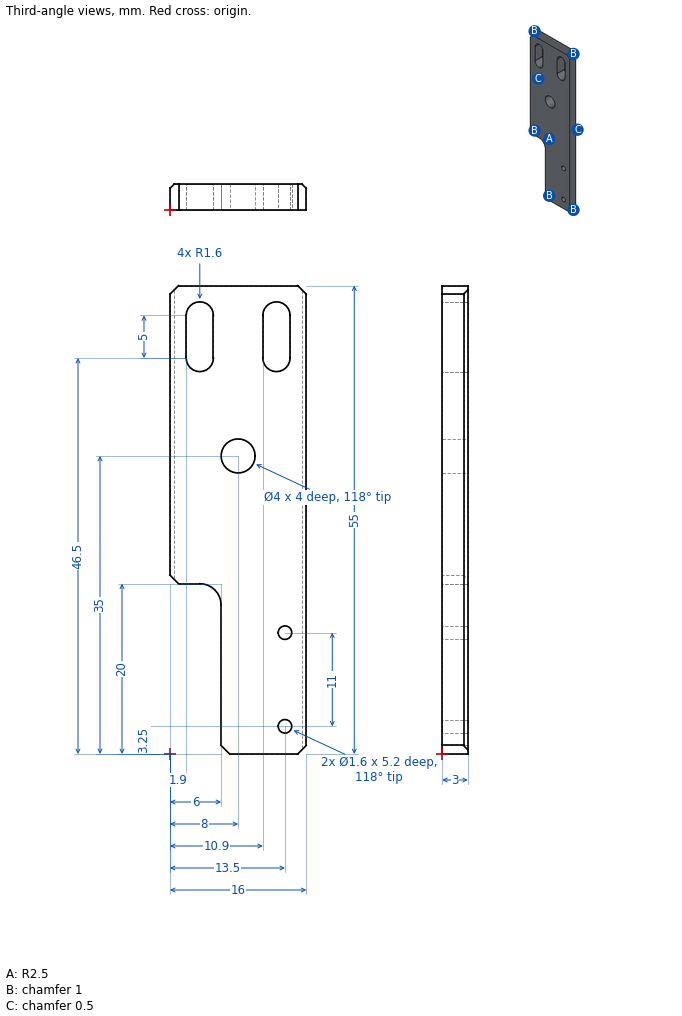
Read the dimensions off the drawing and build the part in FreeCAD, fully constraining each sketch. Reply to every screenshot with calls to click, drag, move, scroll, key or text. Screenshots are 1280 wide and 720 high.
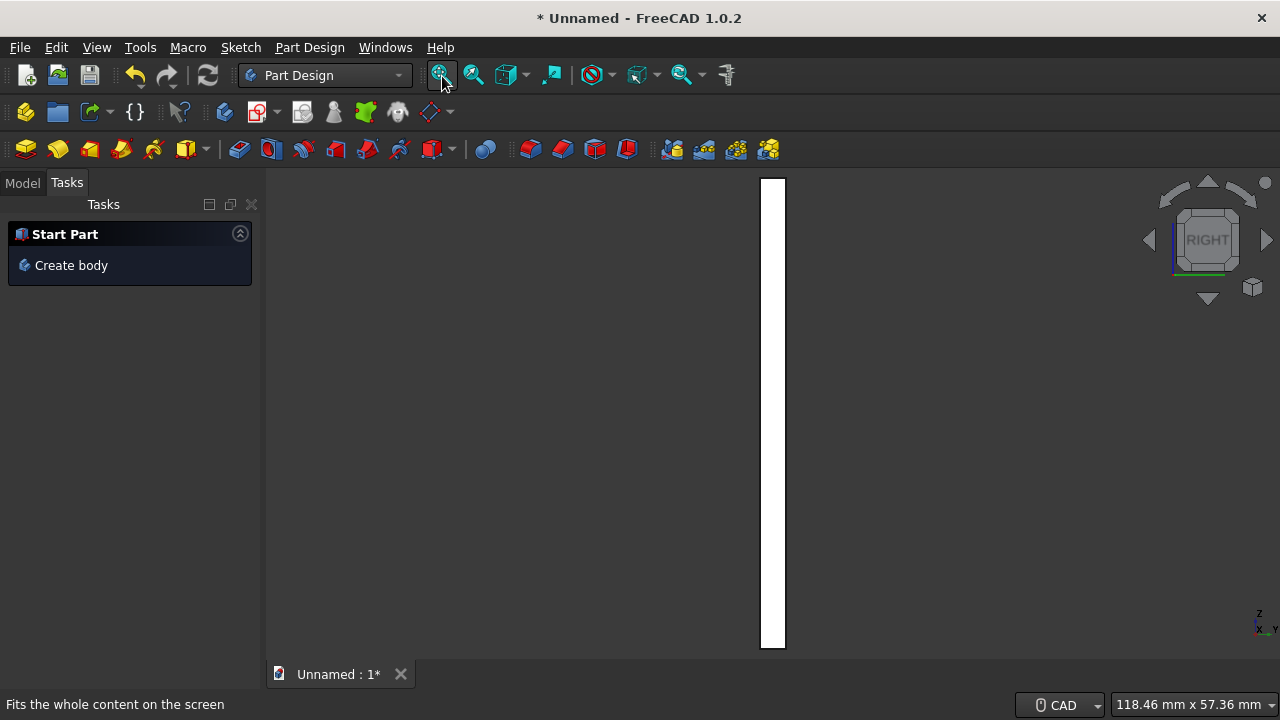
key(5)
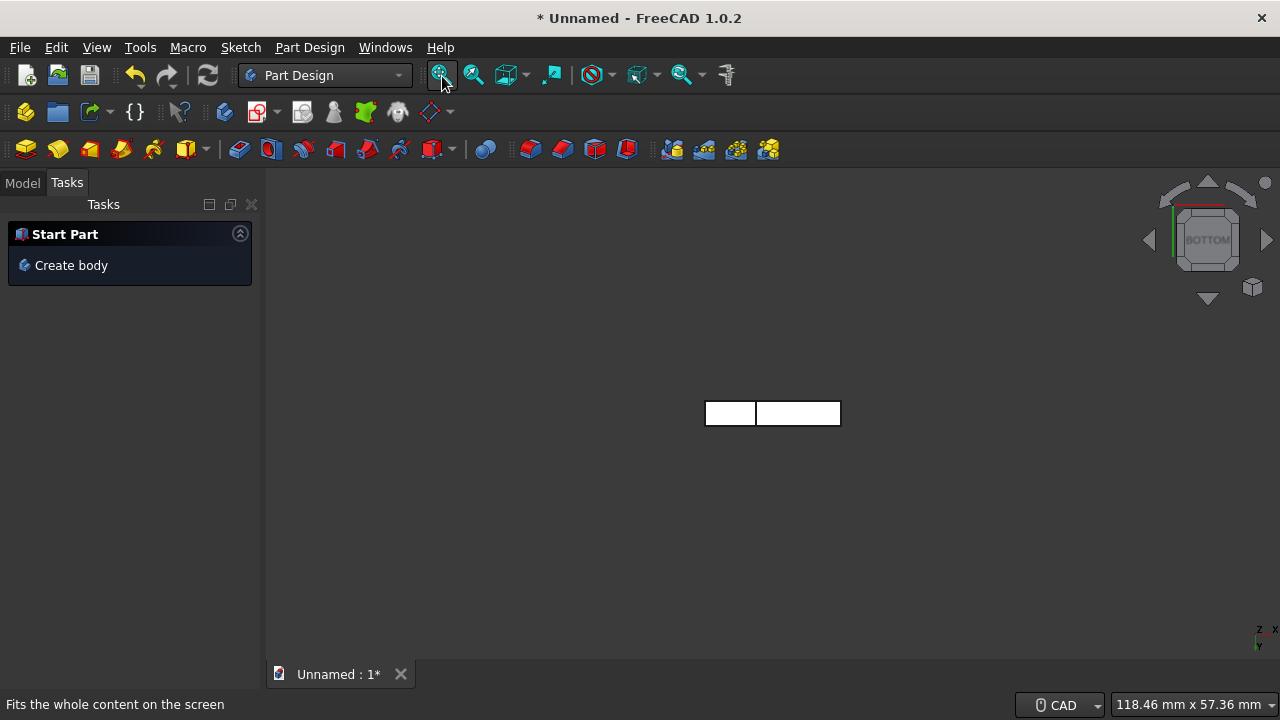
click(442, 76)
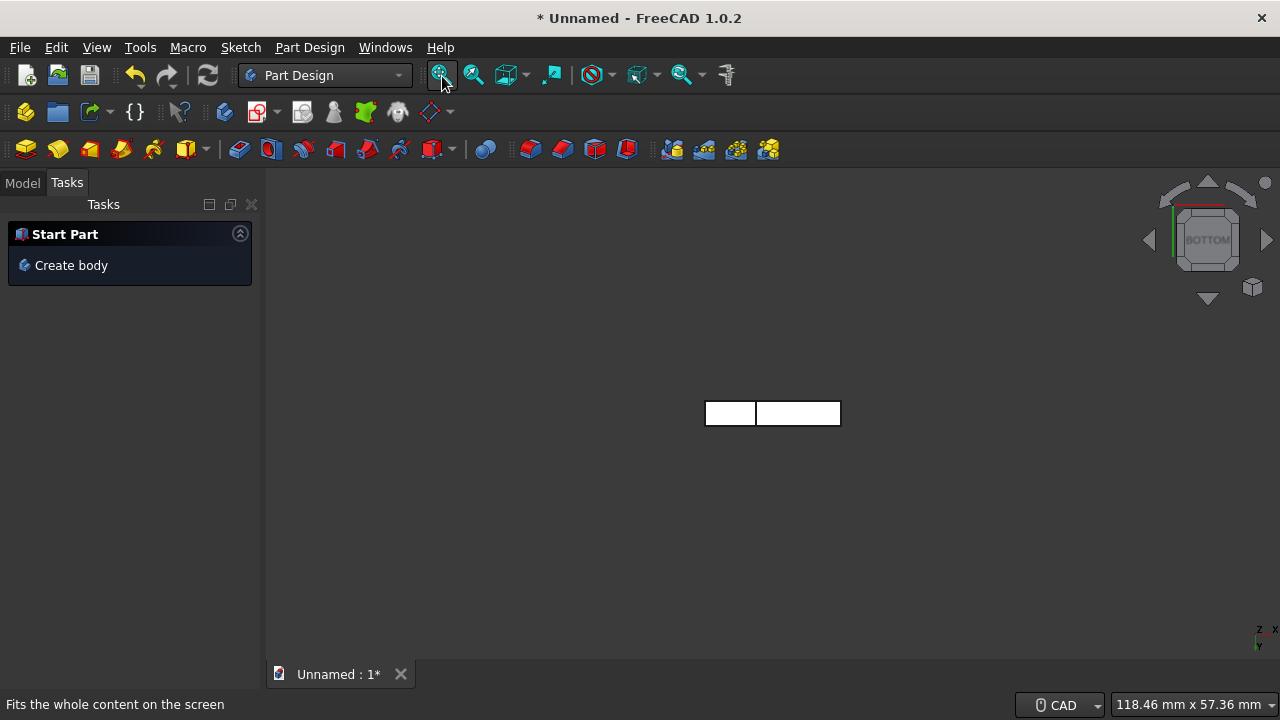
key(4)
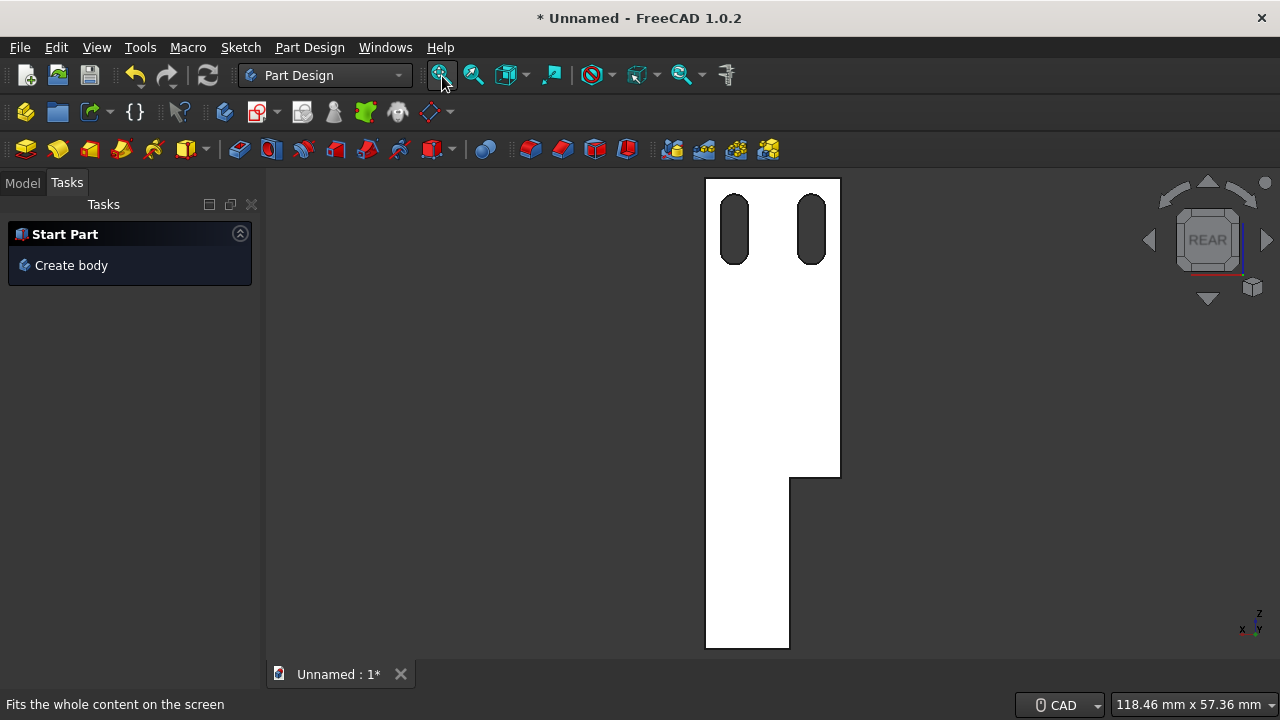
key(6)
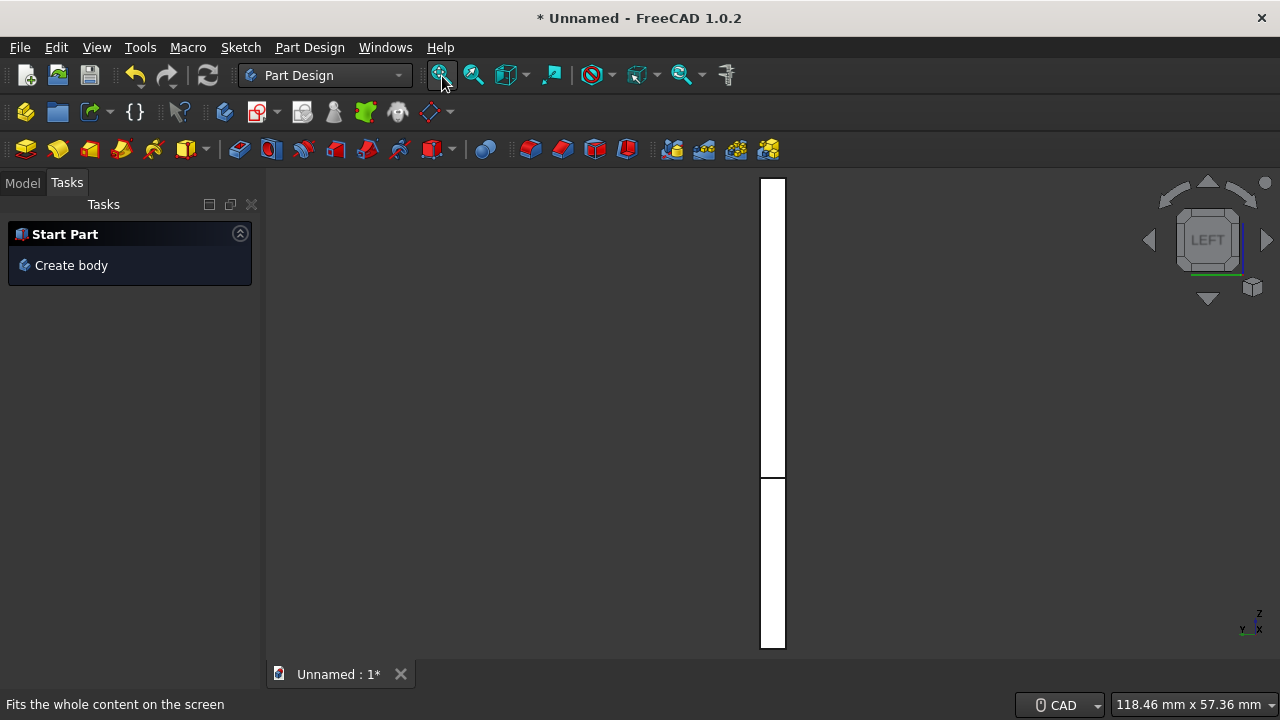
key(v)
key(3)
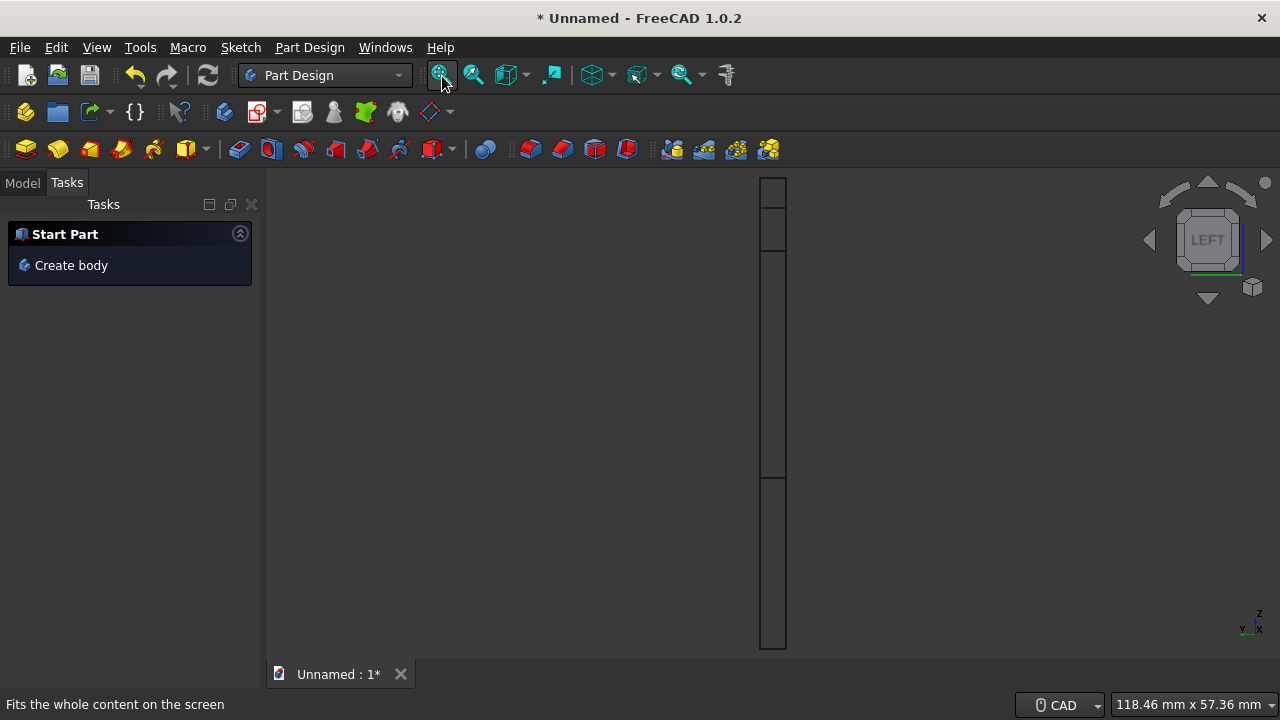
key(0)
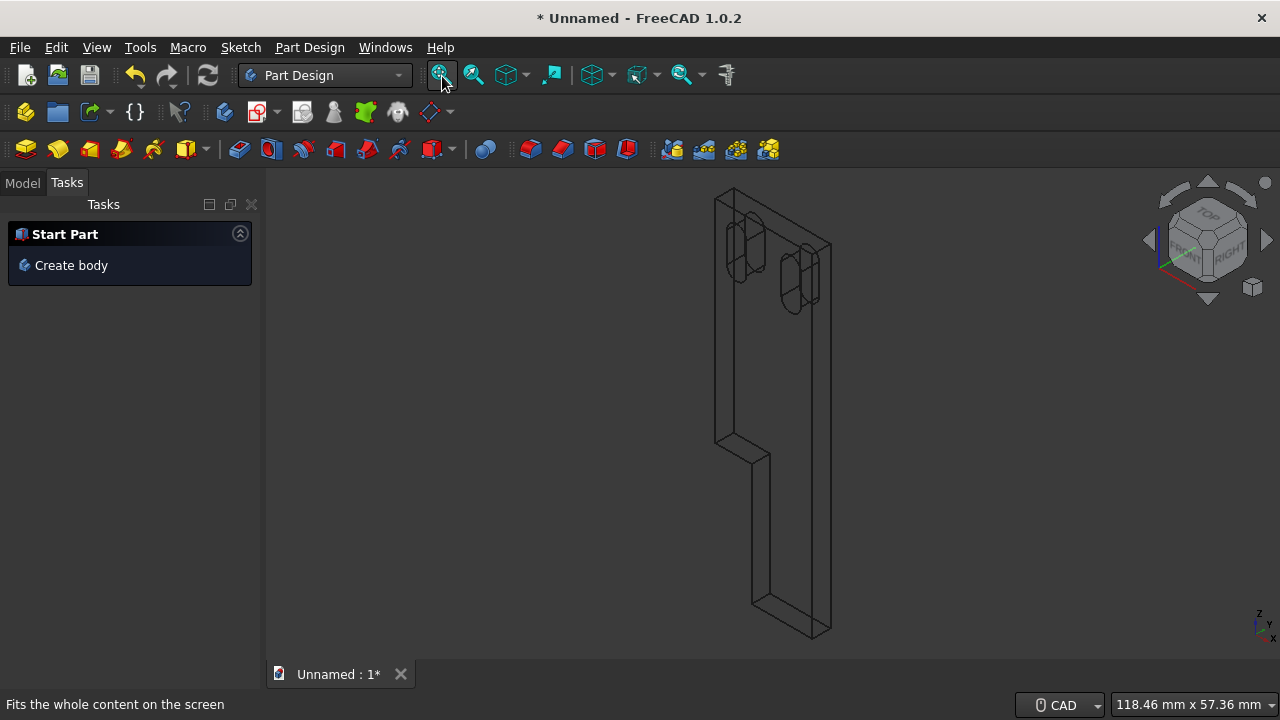
click(761, 458)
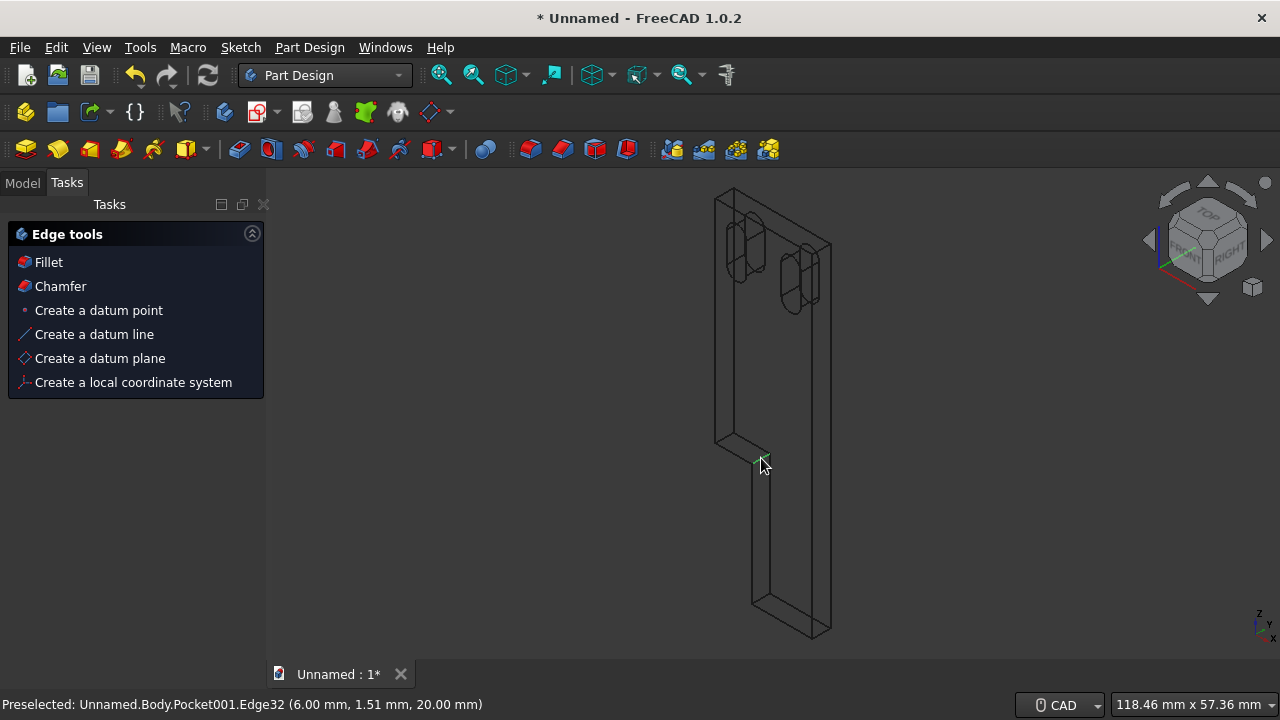
key(v)
key(1)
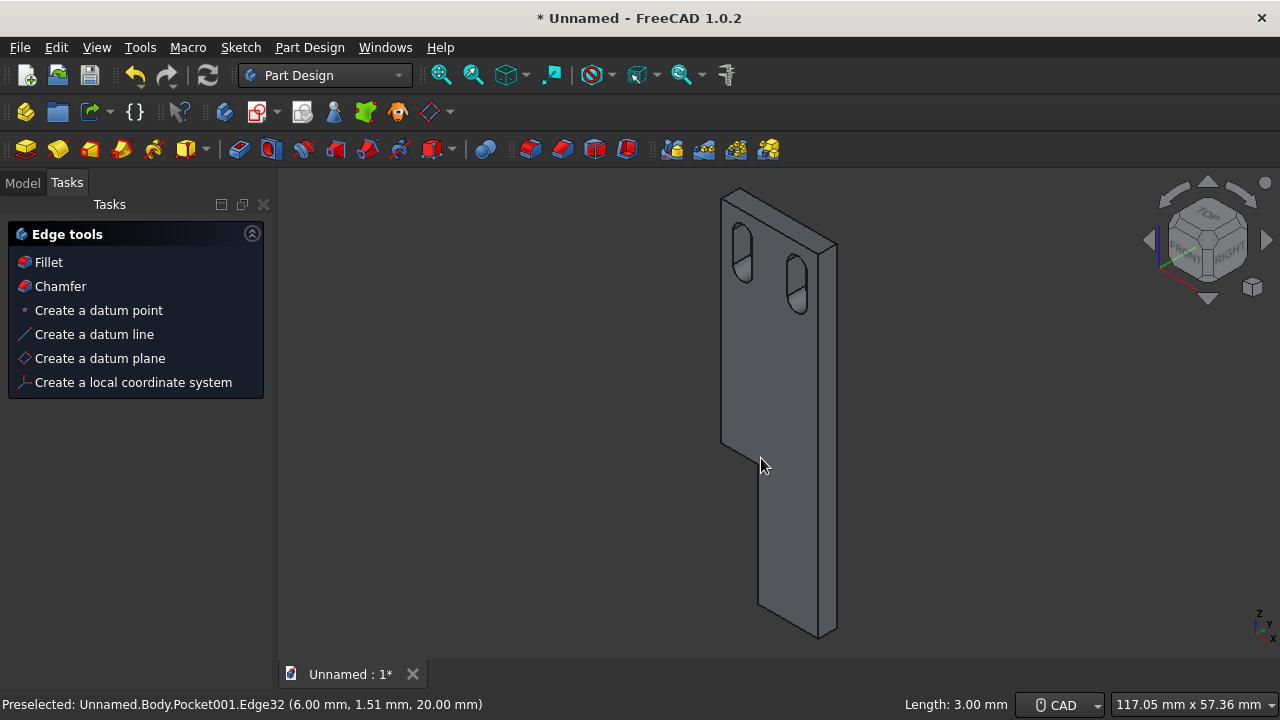
click(532, 150)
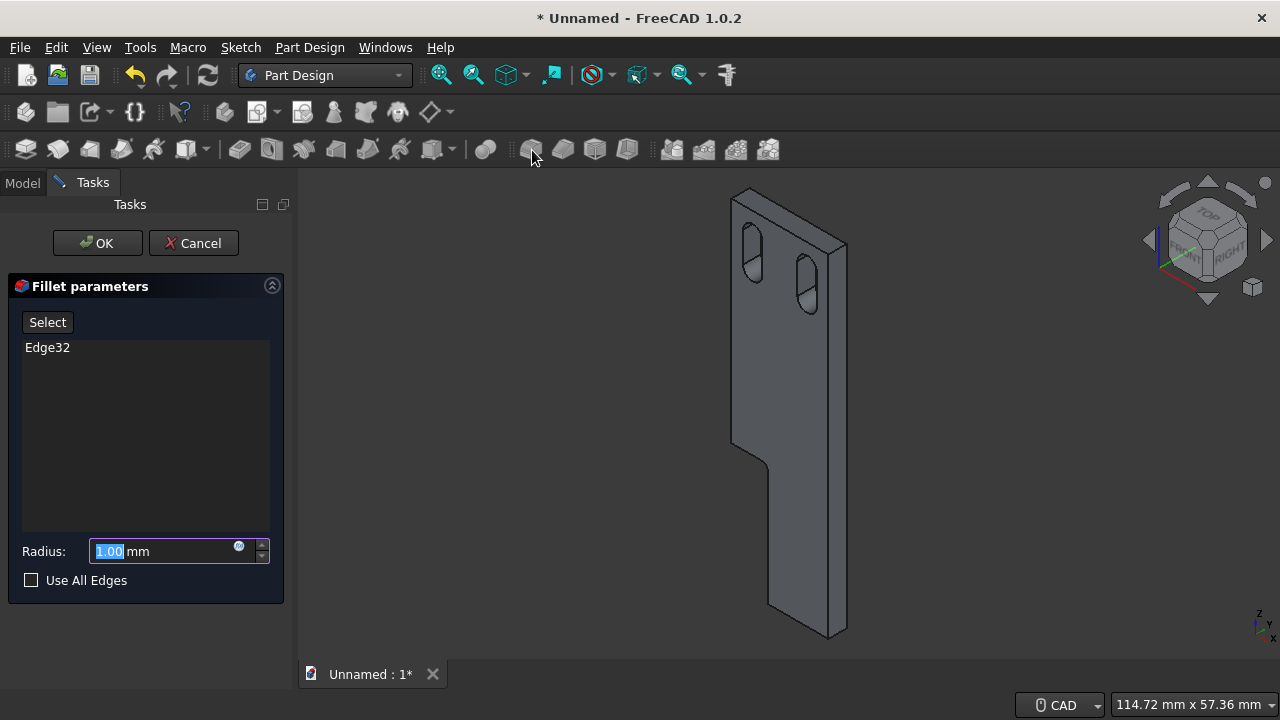
text(2.5)
key(Tab)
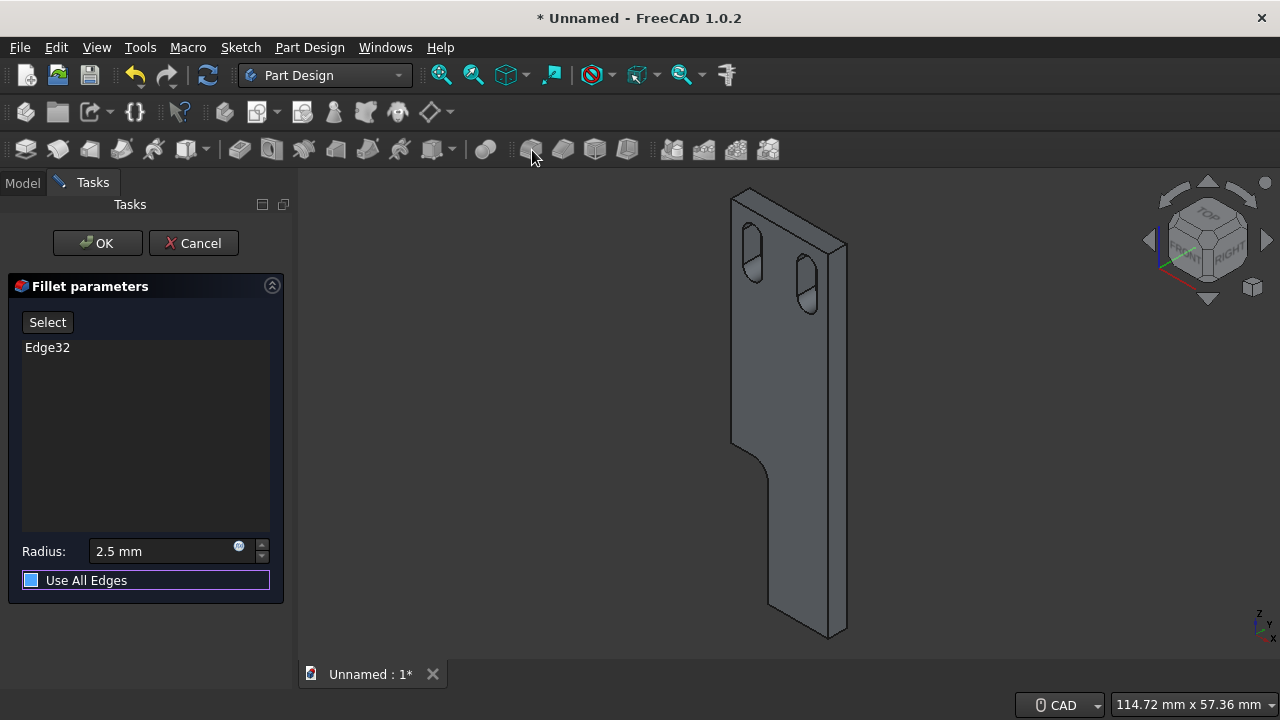
click(98, 243)